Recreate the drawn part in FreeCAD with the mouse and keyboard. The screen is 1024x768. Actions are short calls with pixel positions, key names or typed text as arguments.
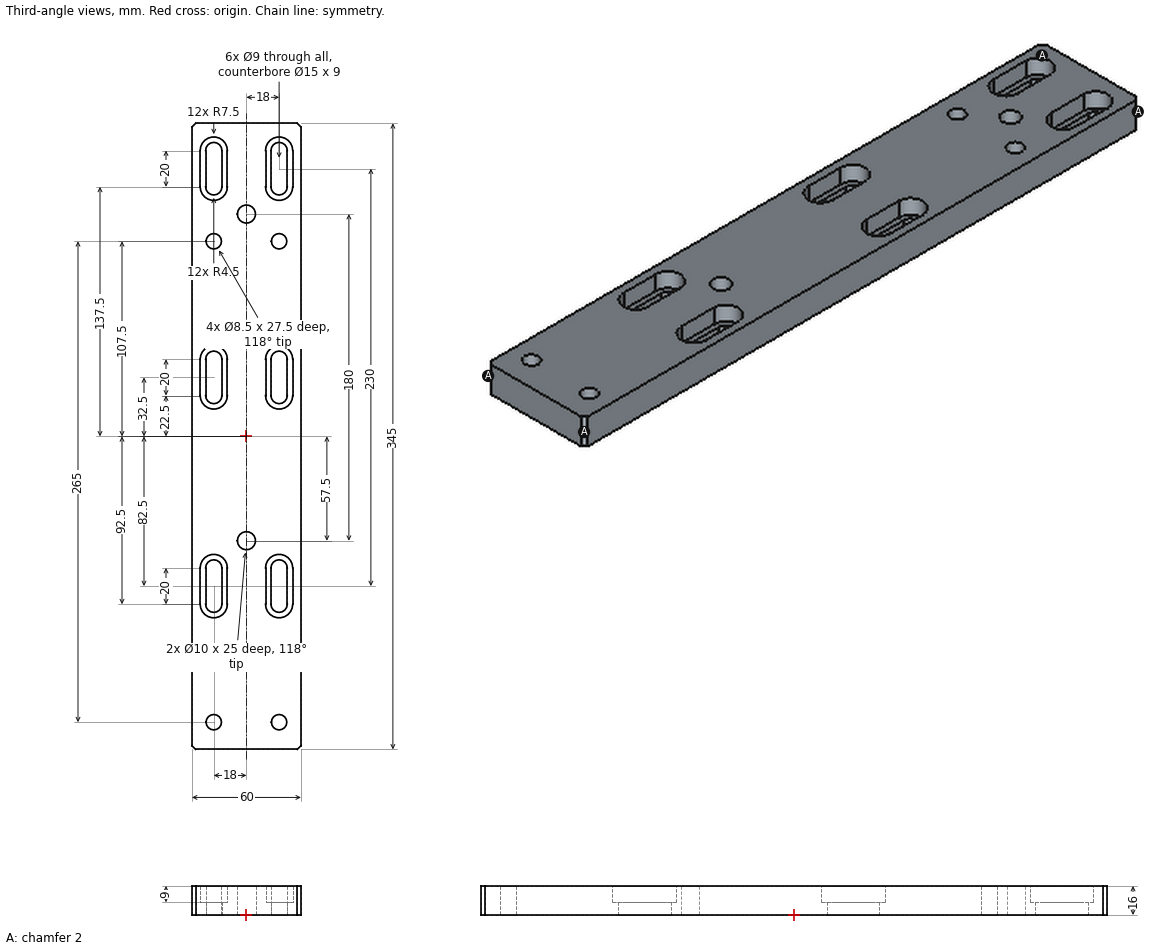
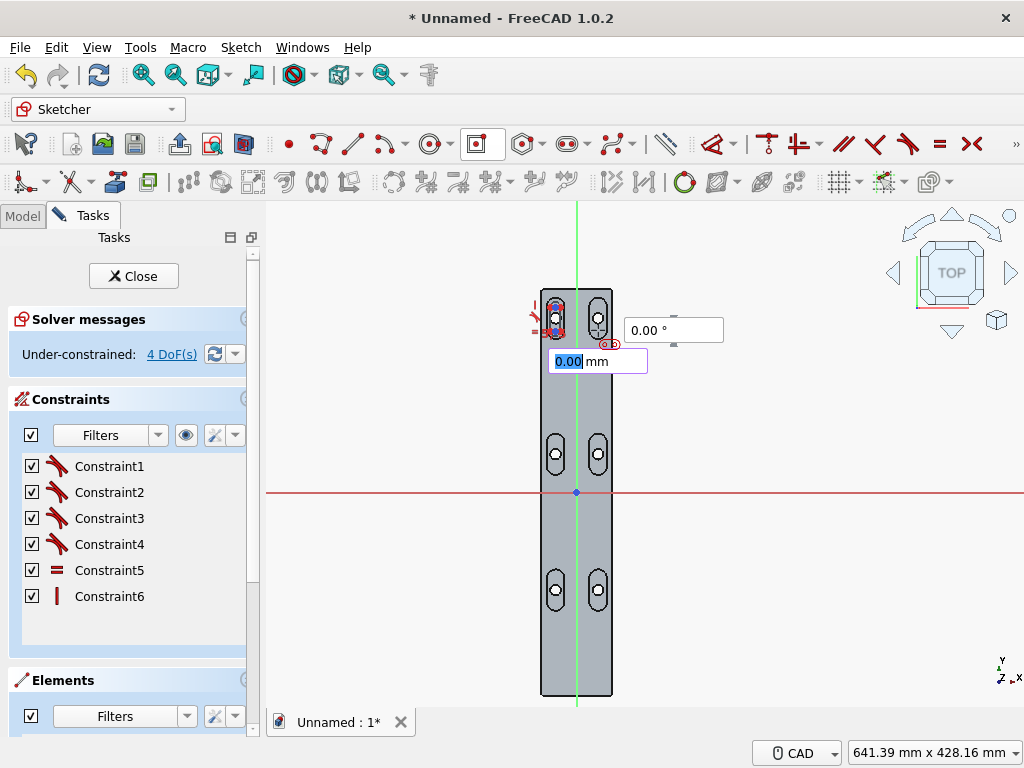
click(598, 306)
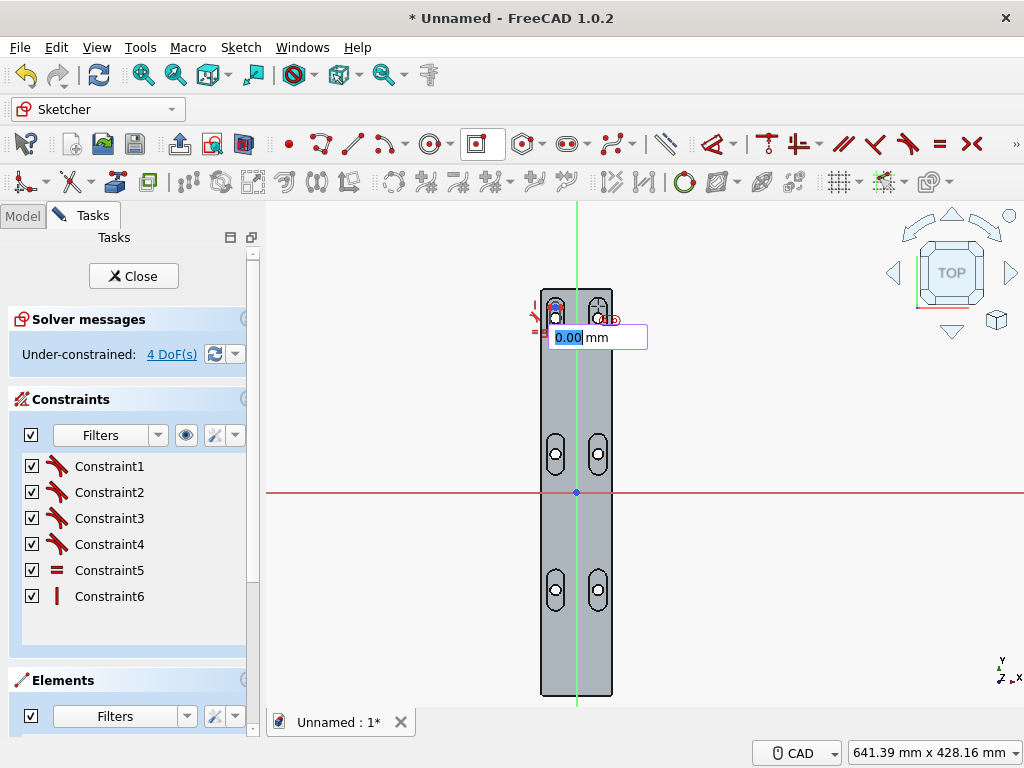
scroll(593, 318, up, 6)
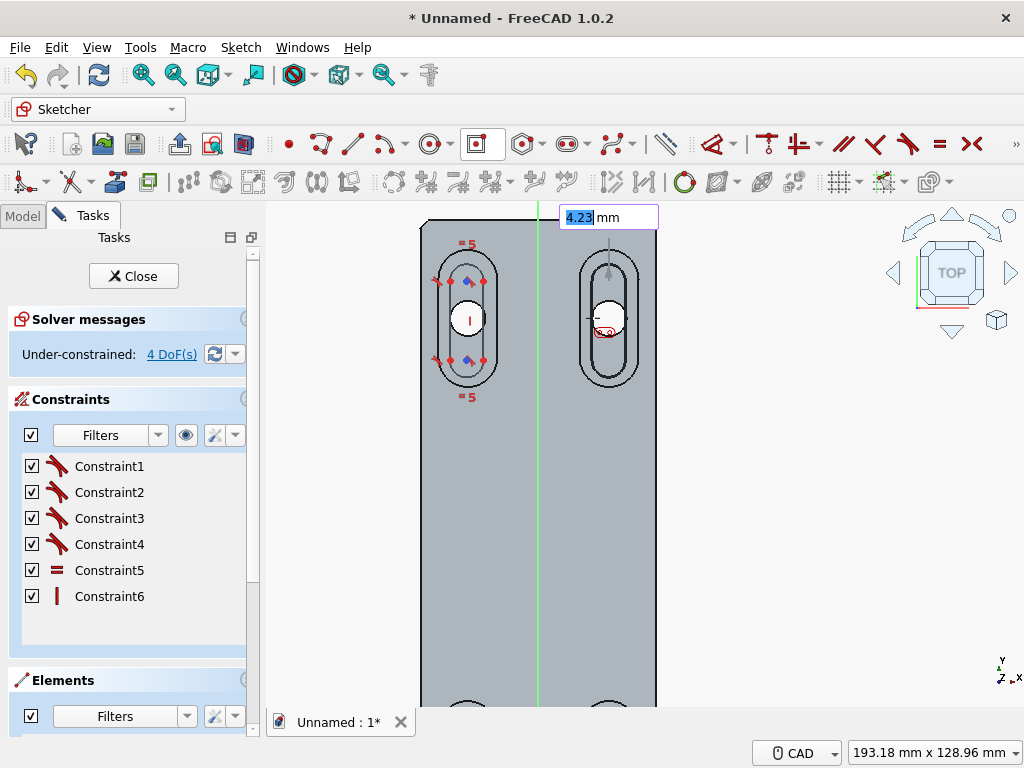
click(591, 318)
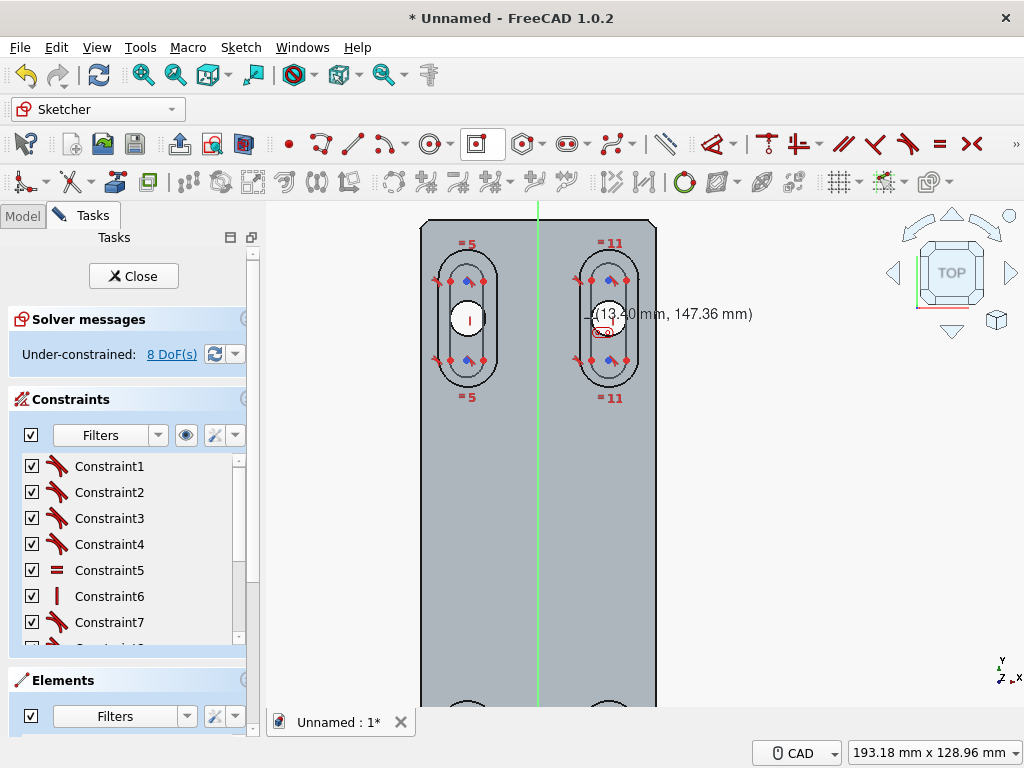
scroll(593, 318, down, 6)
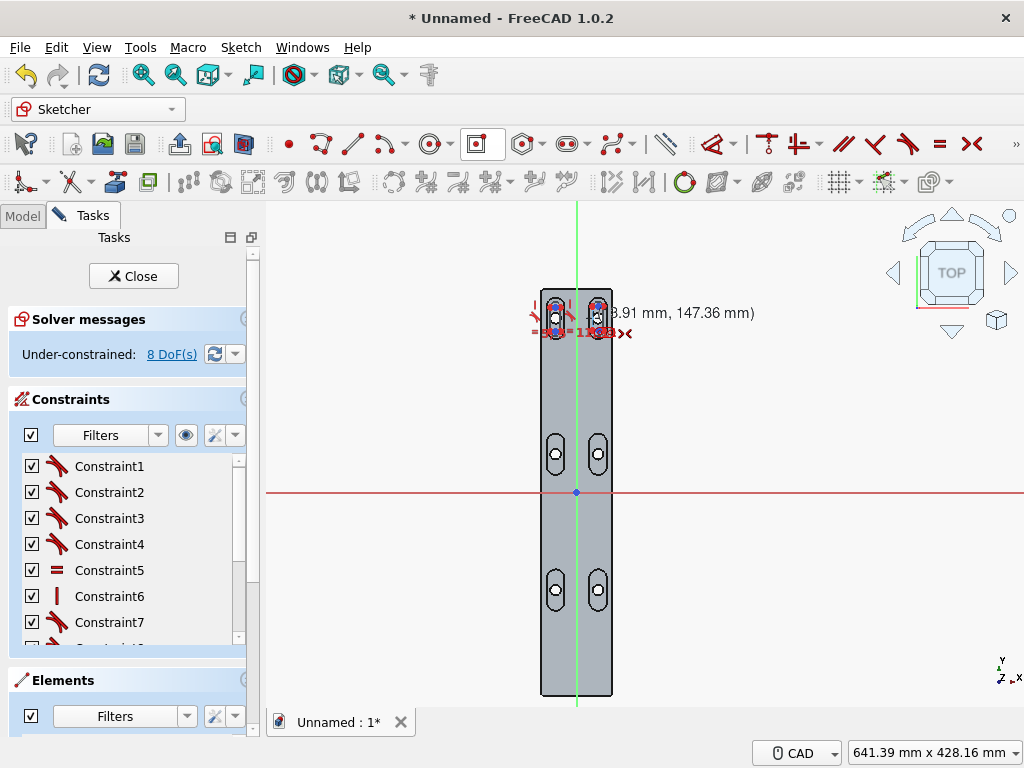
scroll(556, 466, up, 8)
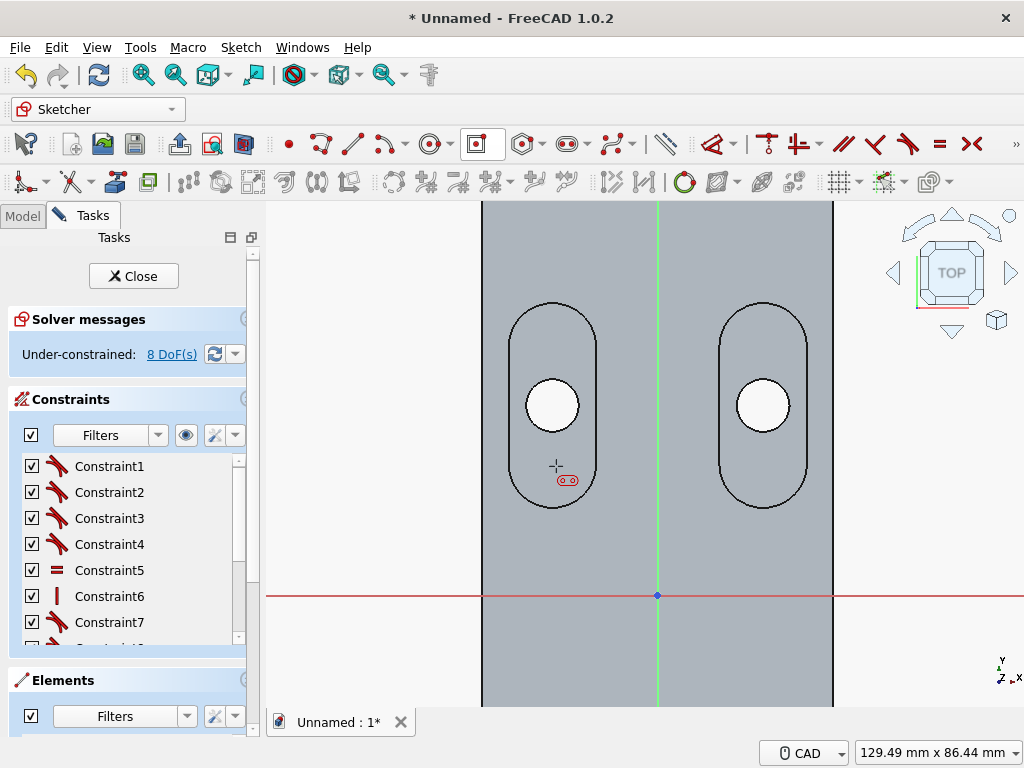
scroll(556, 466, down, 8)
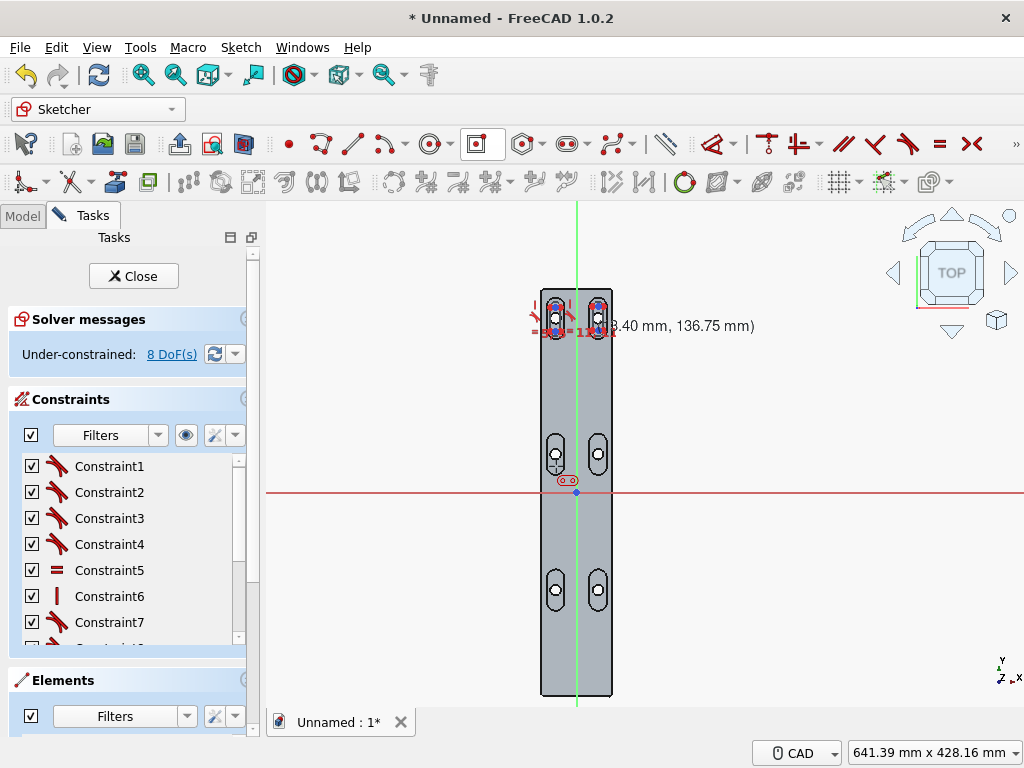
click(556, 466)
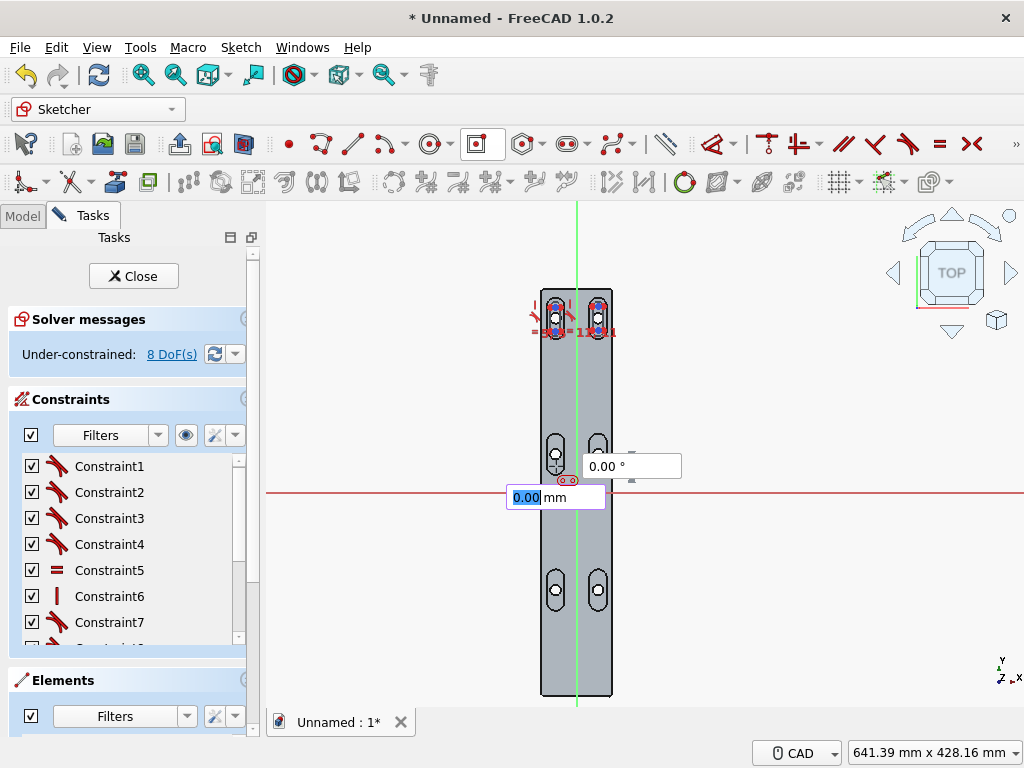
click(556, 442)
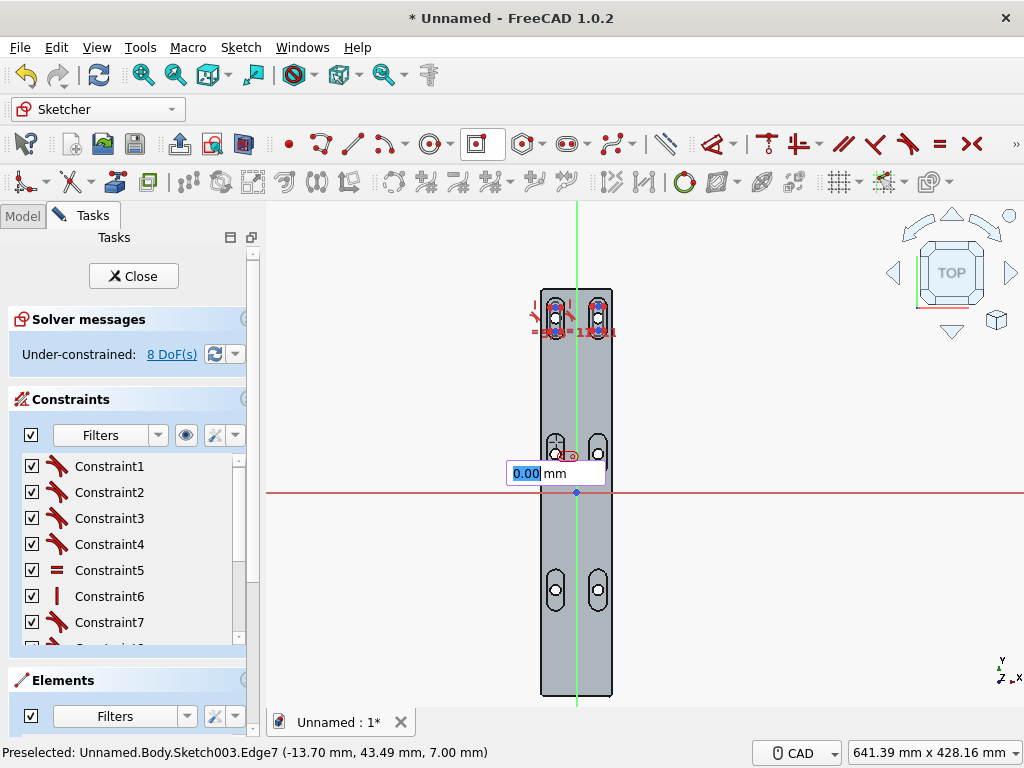
scroll(550, 454, up, 6)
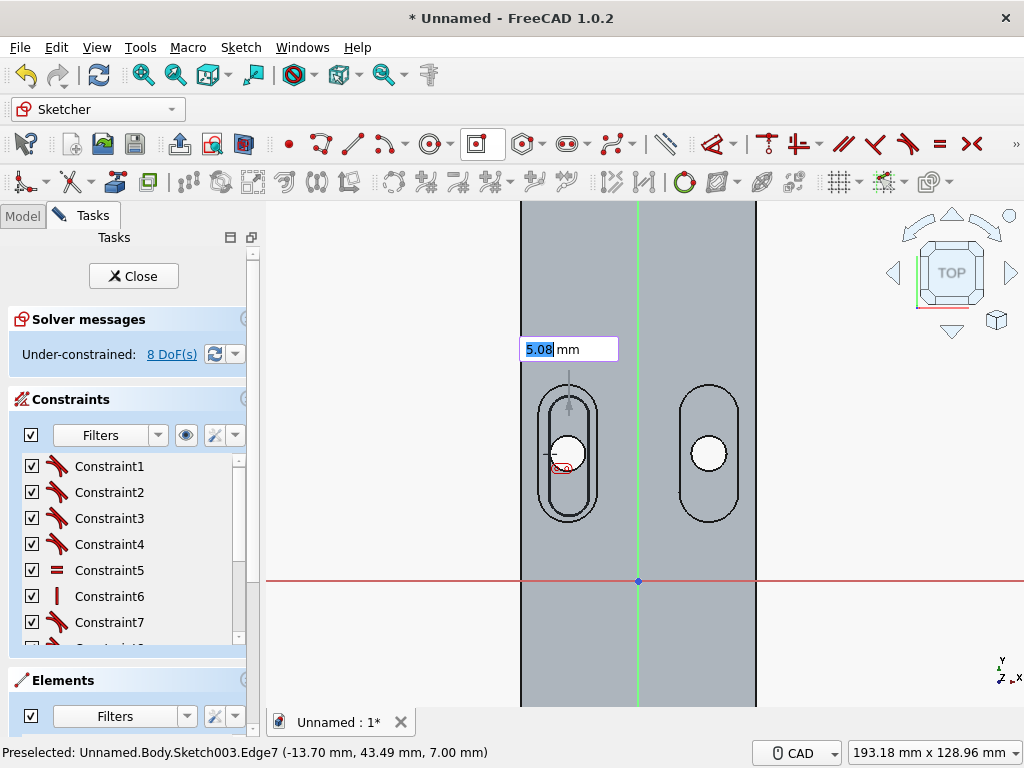
click(550, 454)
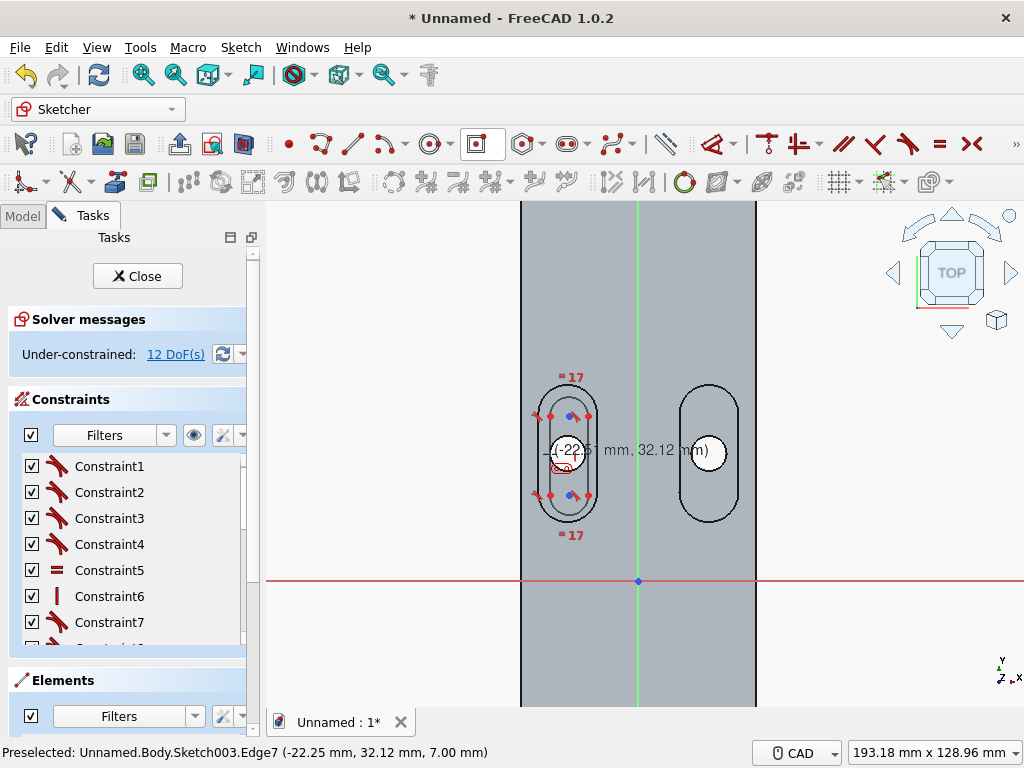
scroll(709, 493, up, 2)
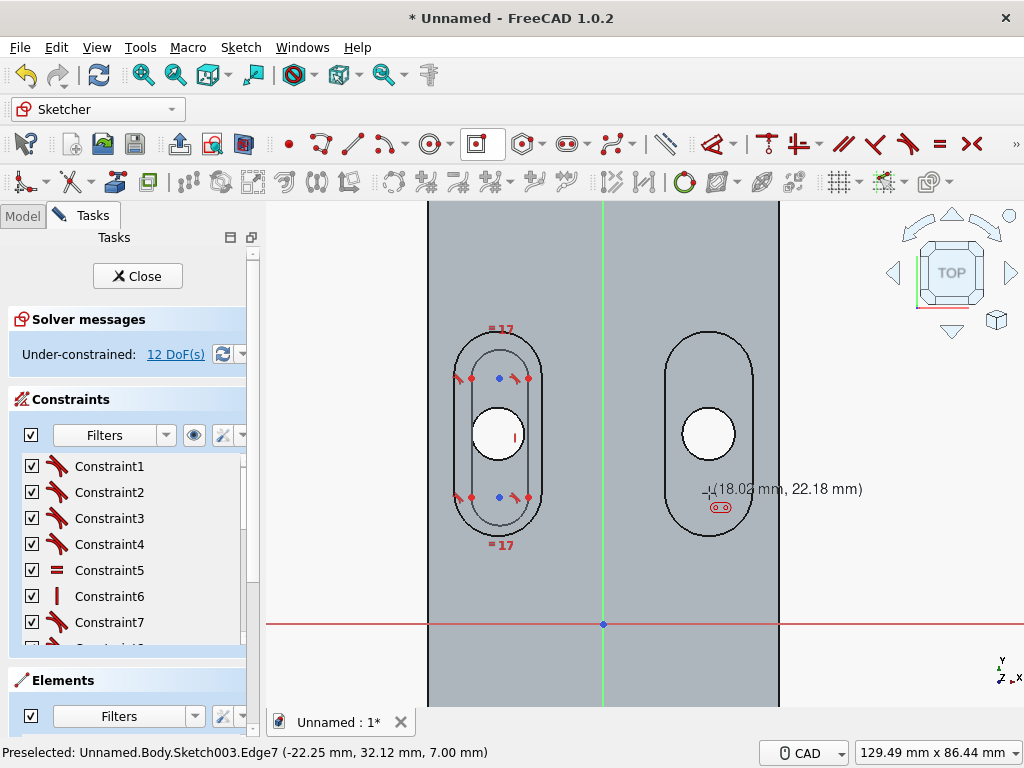
scroll(570, 459, down, 8)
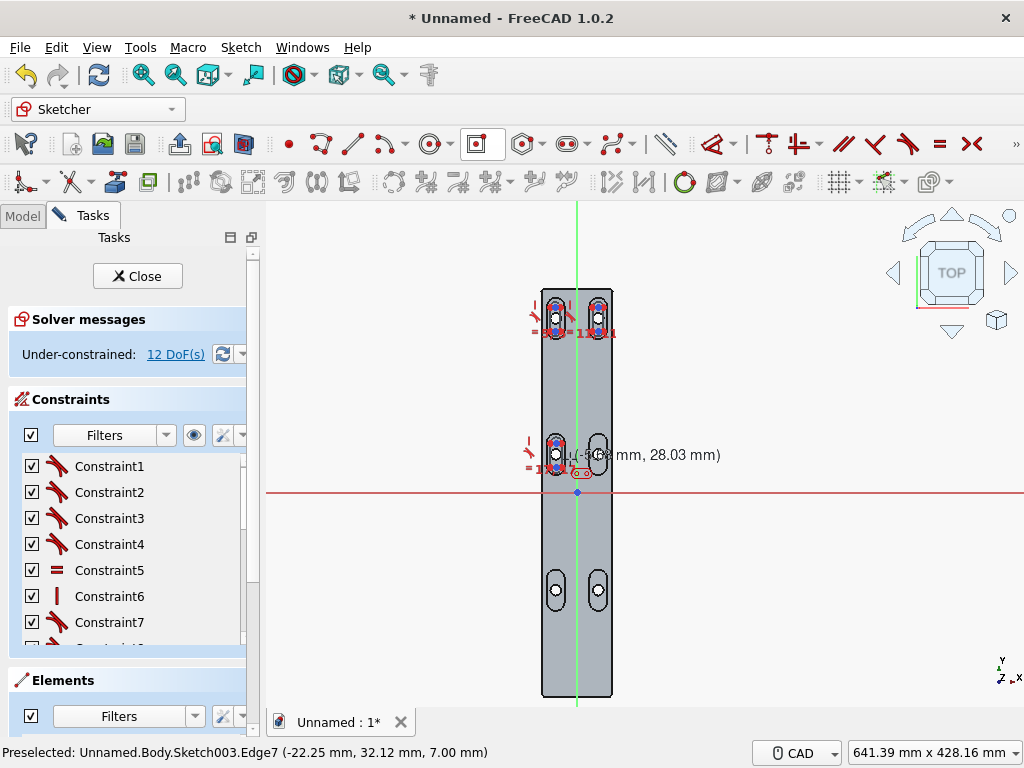
click(598, 466)